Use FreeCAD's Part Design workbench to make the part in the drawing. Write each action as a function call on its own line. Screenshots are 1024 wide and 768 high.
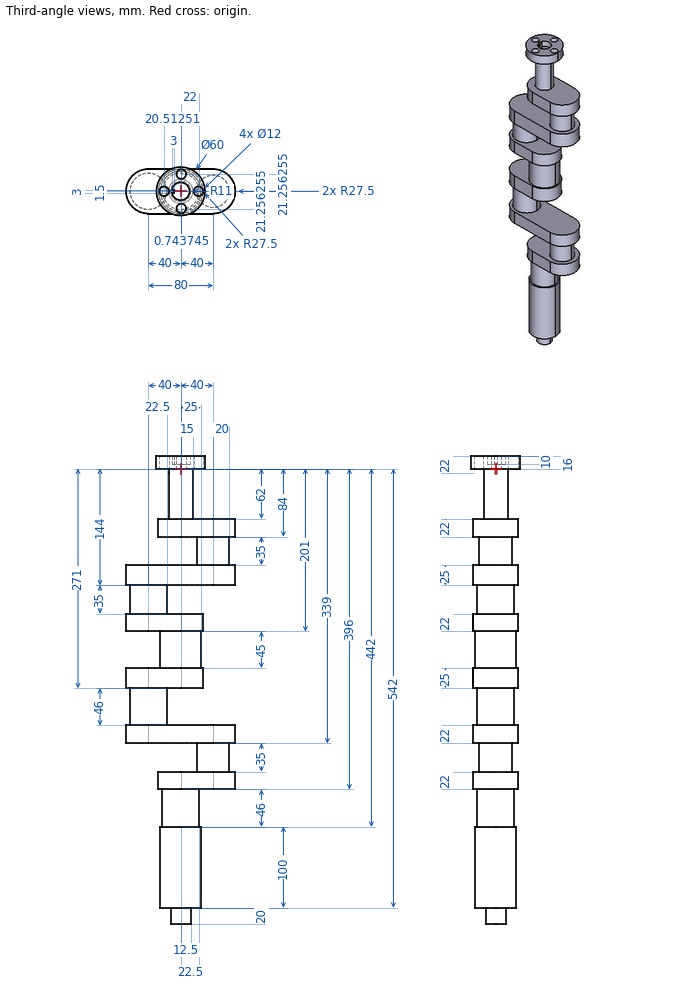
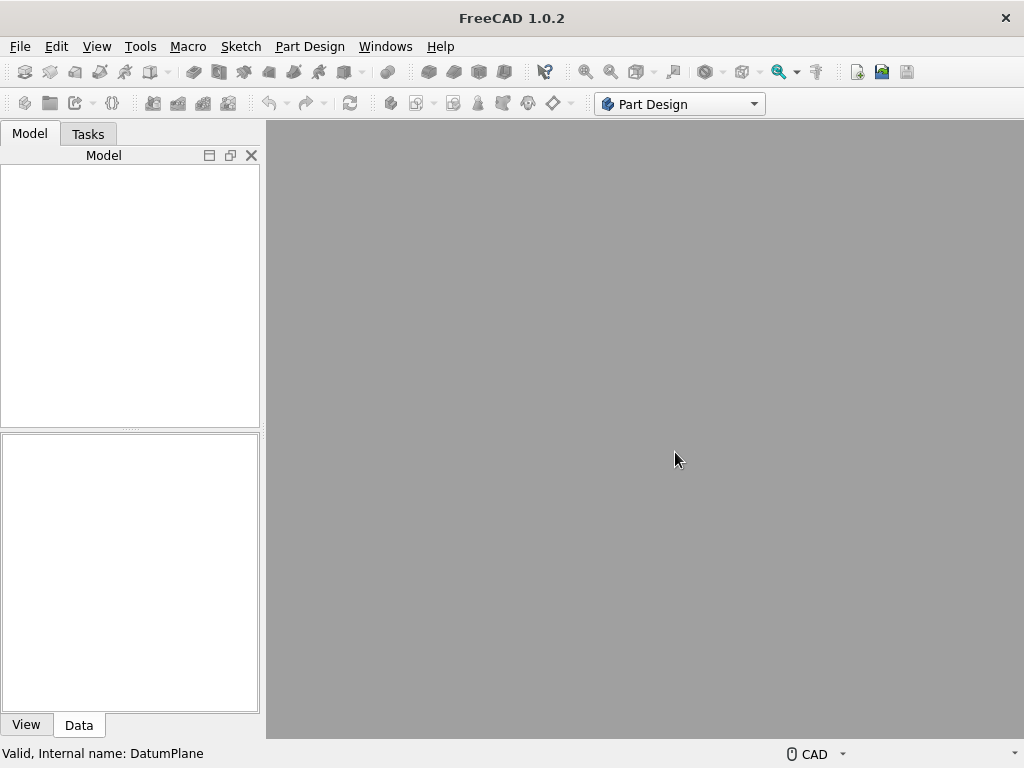
key(ctrl+n)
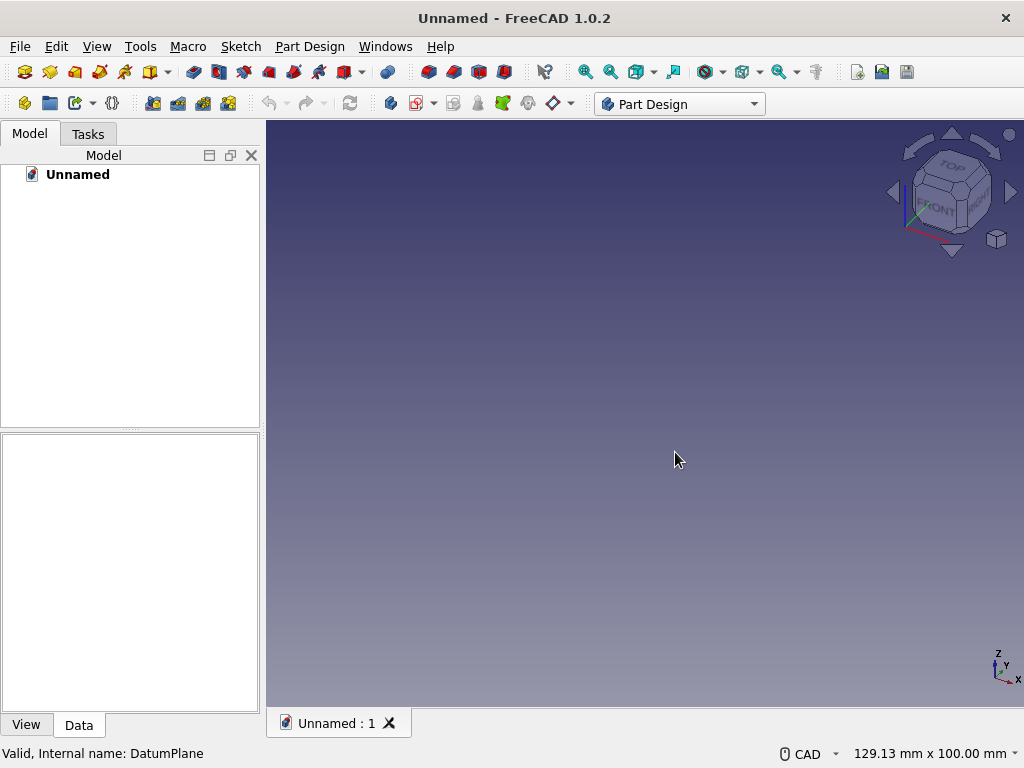
click(416, 104)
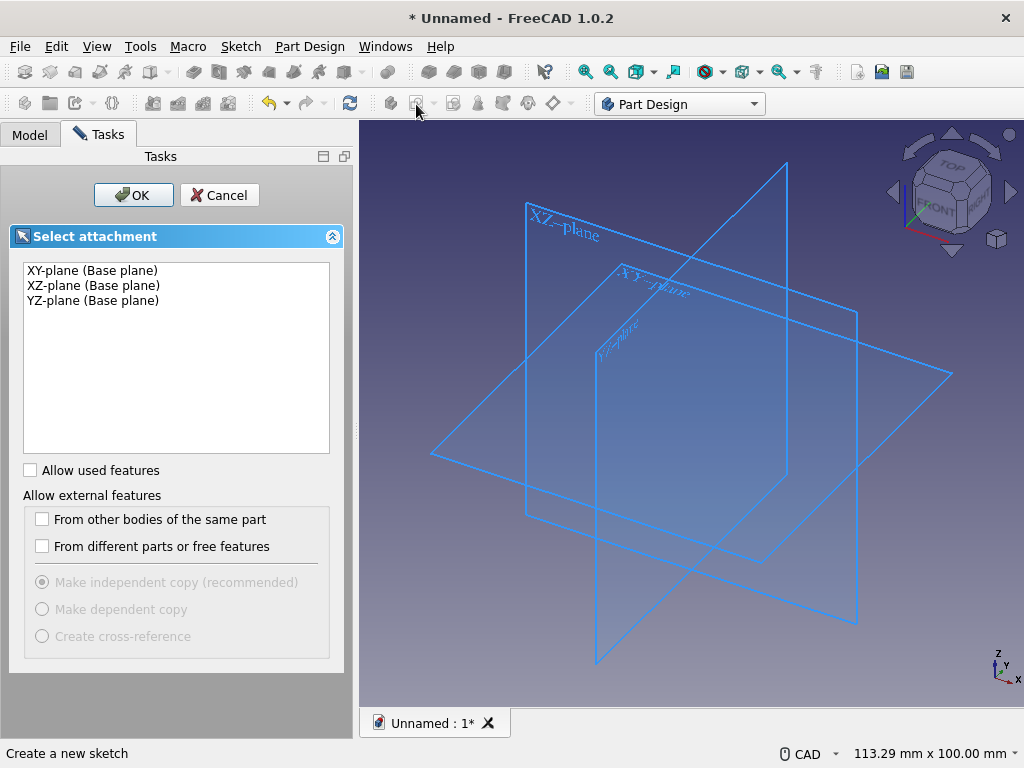
click(84, 270)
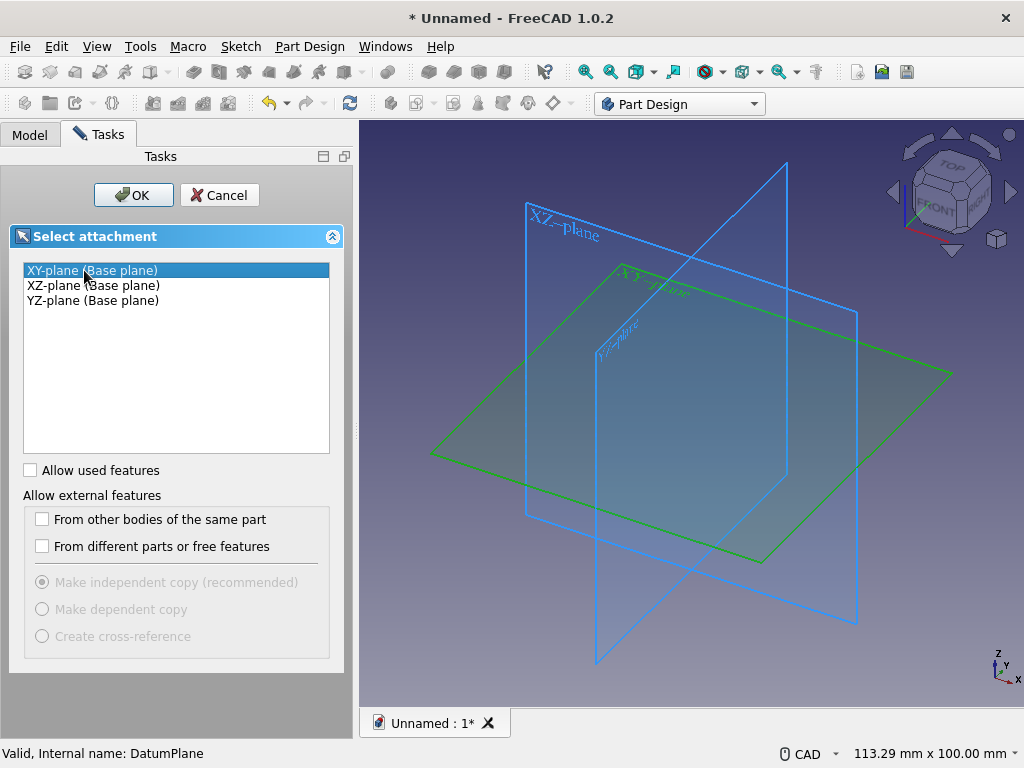
click(134, 195)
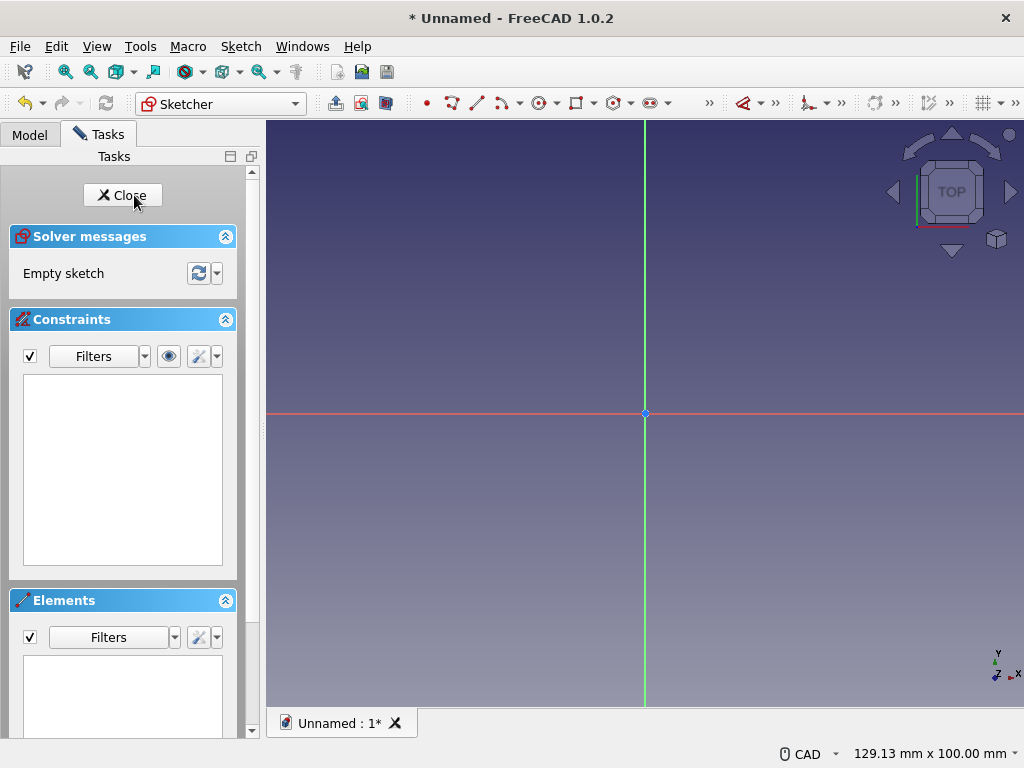
key(g)
key(c)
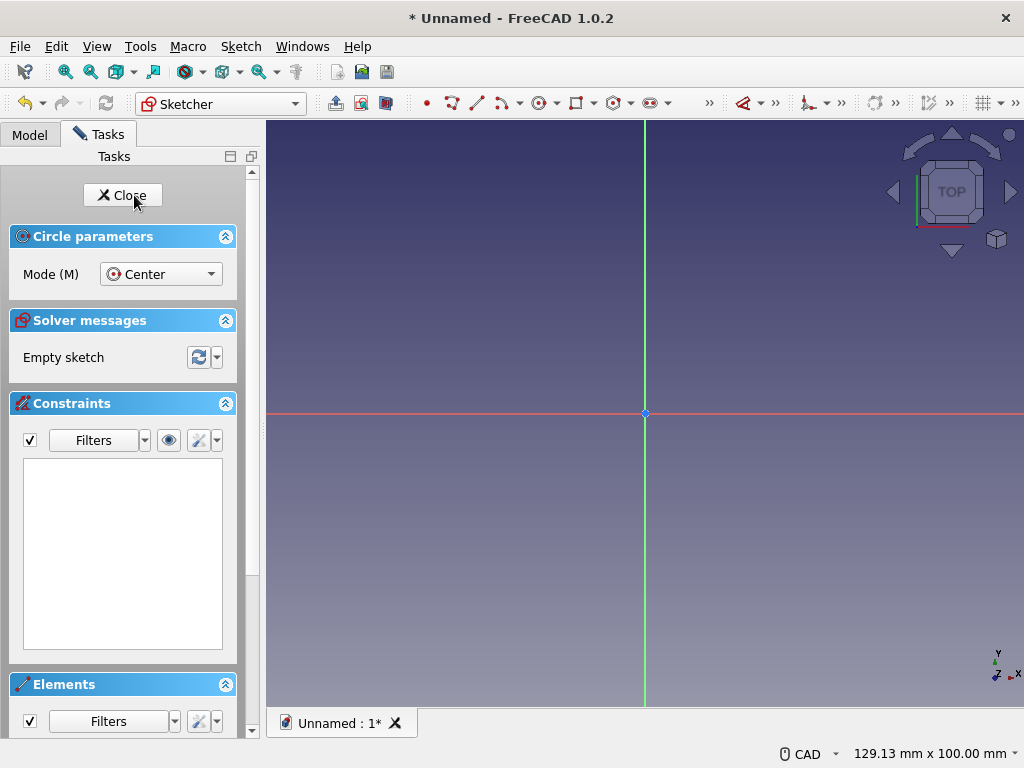
click(645, 414)
move(770, 289)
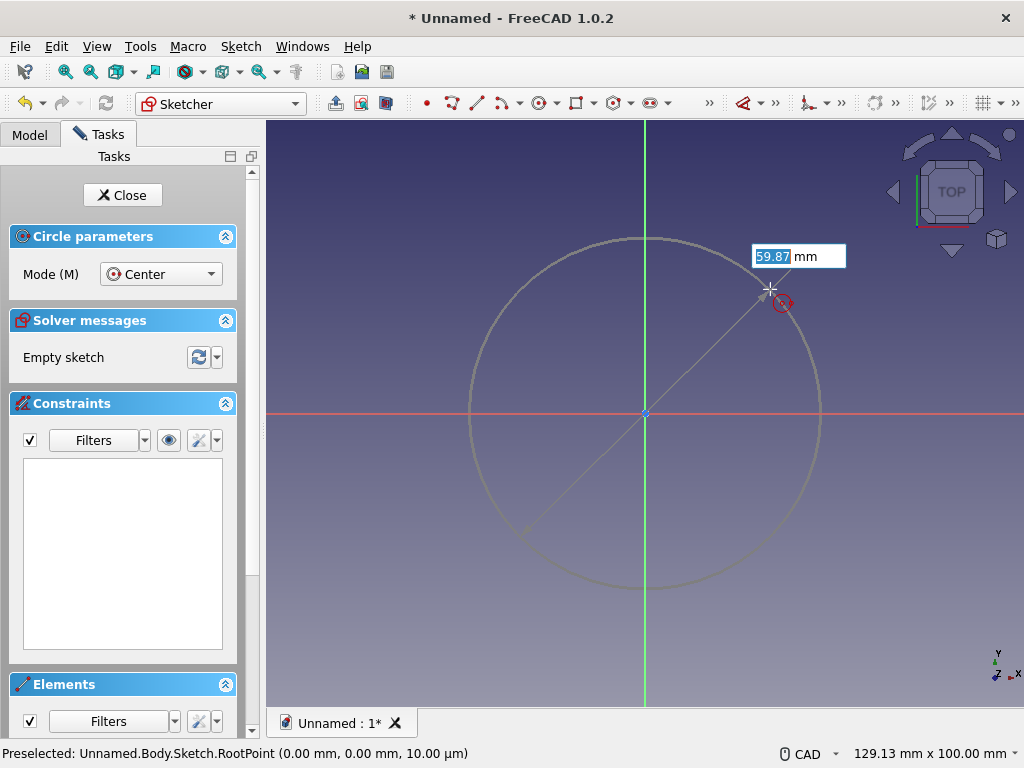
text(60)
key(Return)
key(Escape)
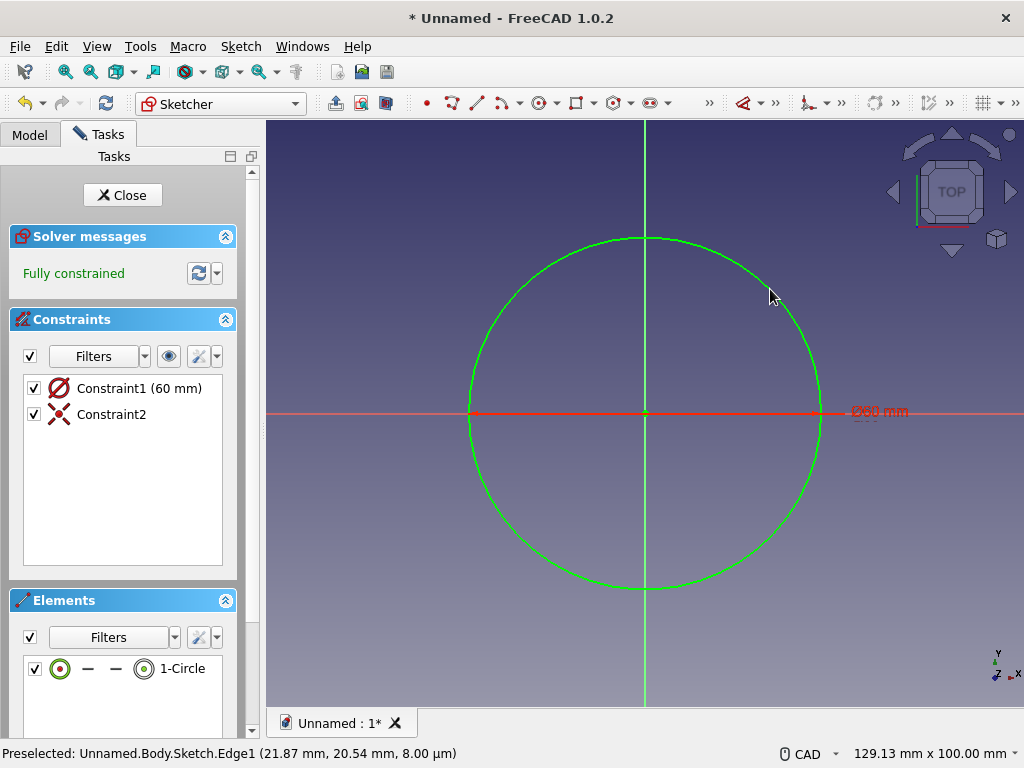
click(123, 195)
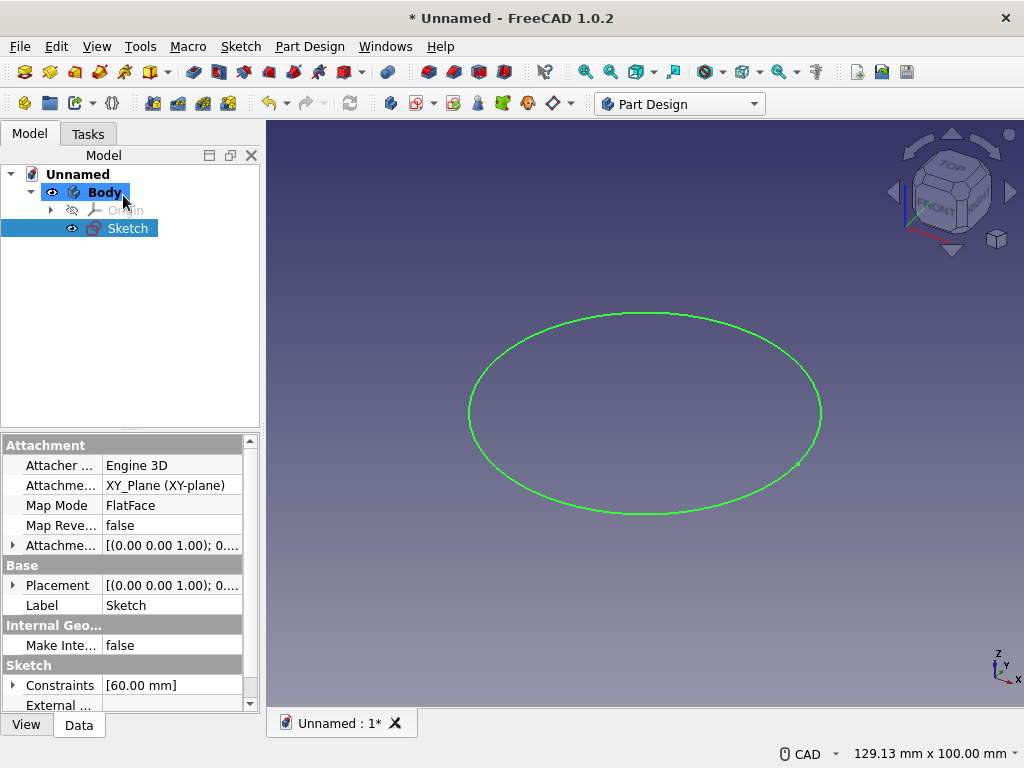
click(25, 72)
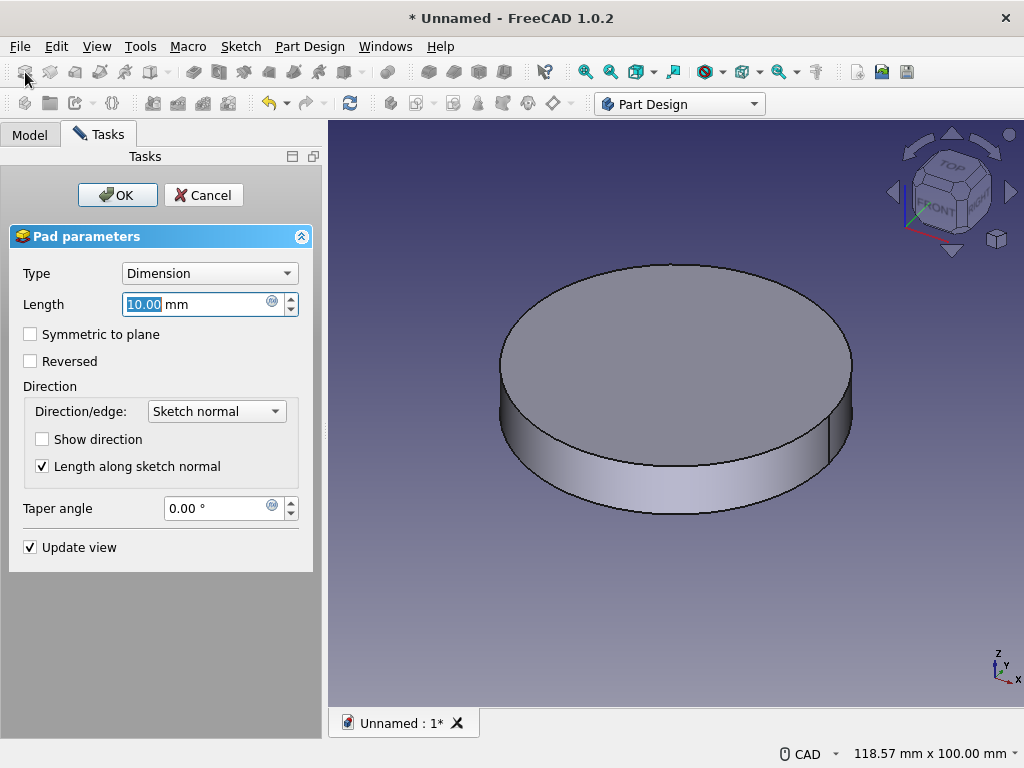
text(16)
key(Tab)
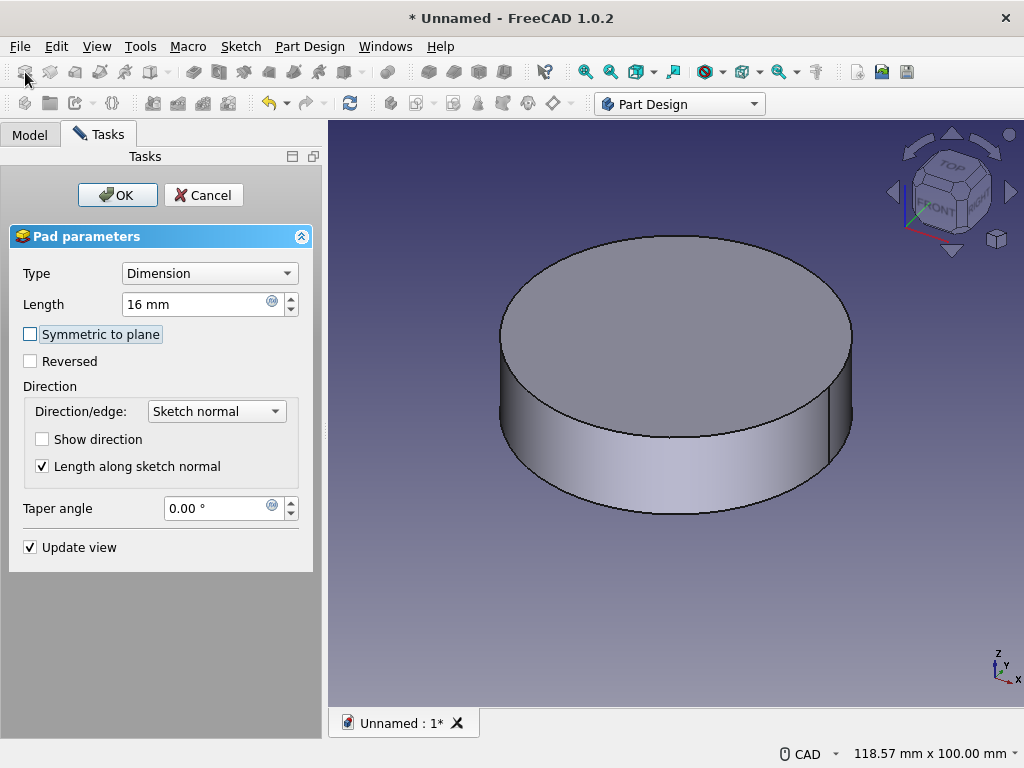
click(118, 195)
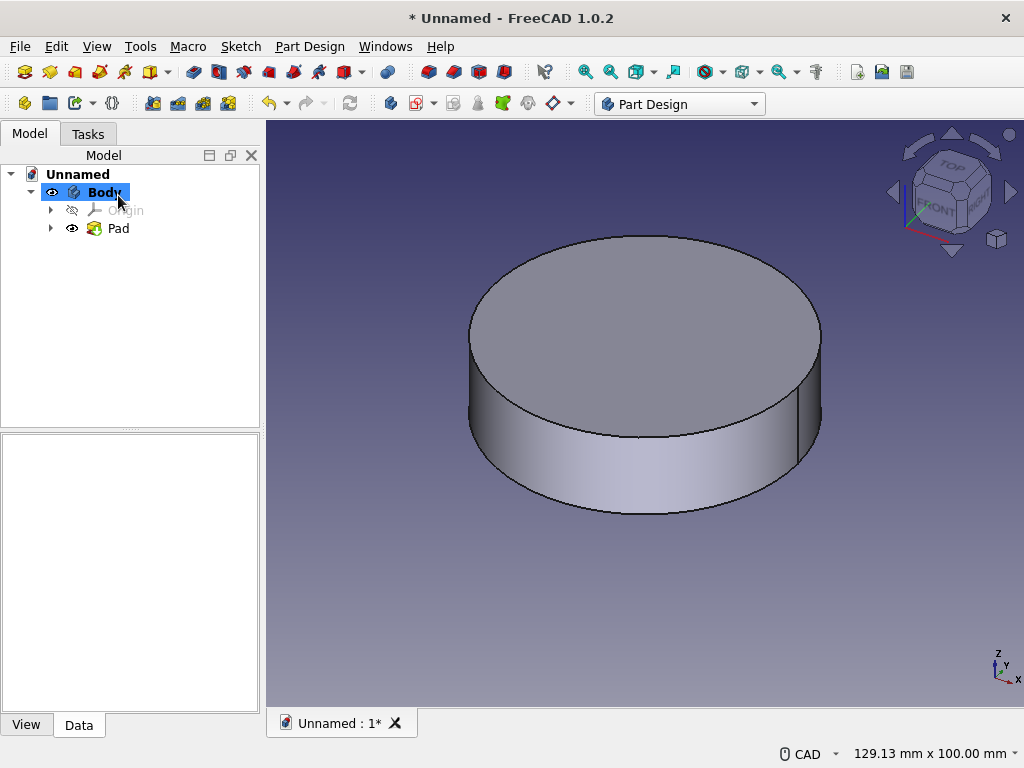
click(416, 104)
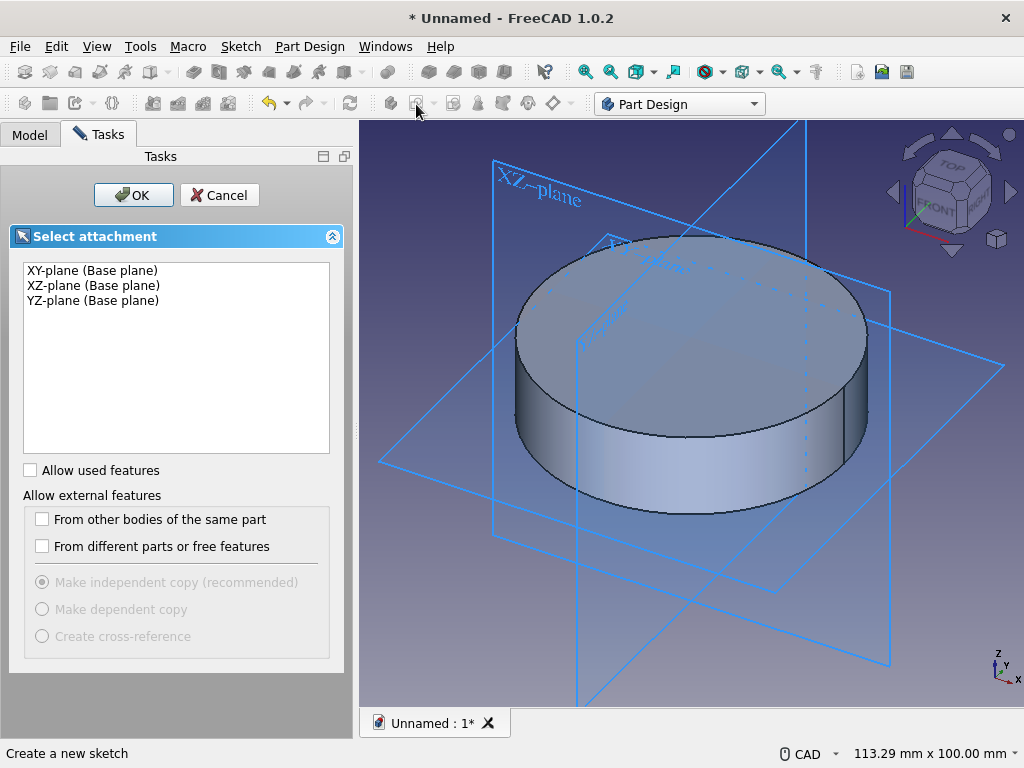
click(84, 286)